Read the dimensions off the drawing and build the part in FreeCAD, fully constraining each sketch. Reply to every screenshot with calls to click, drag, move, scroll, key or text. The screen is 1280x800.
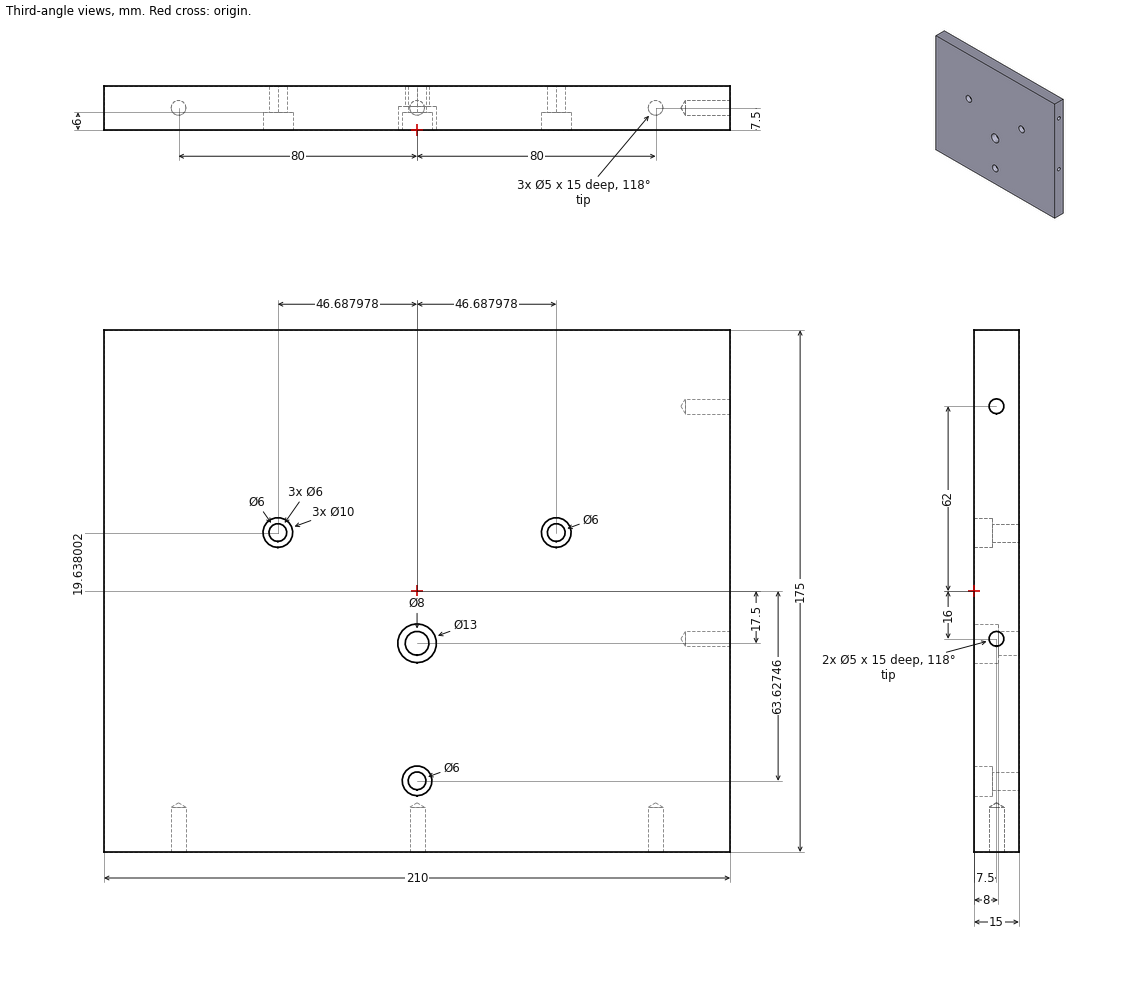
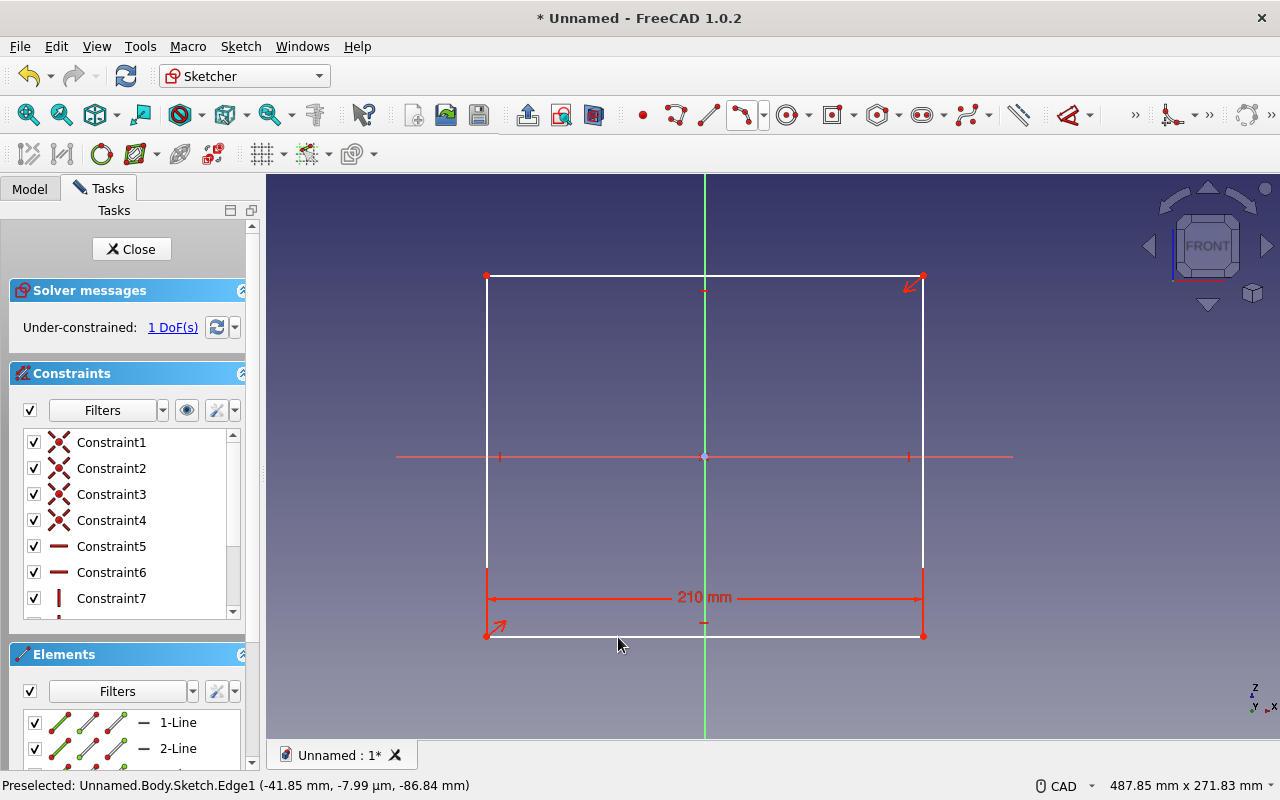
click(923, 529)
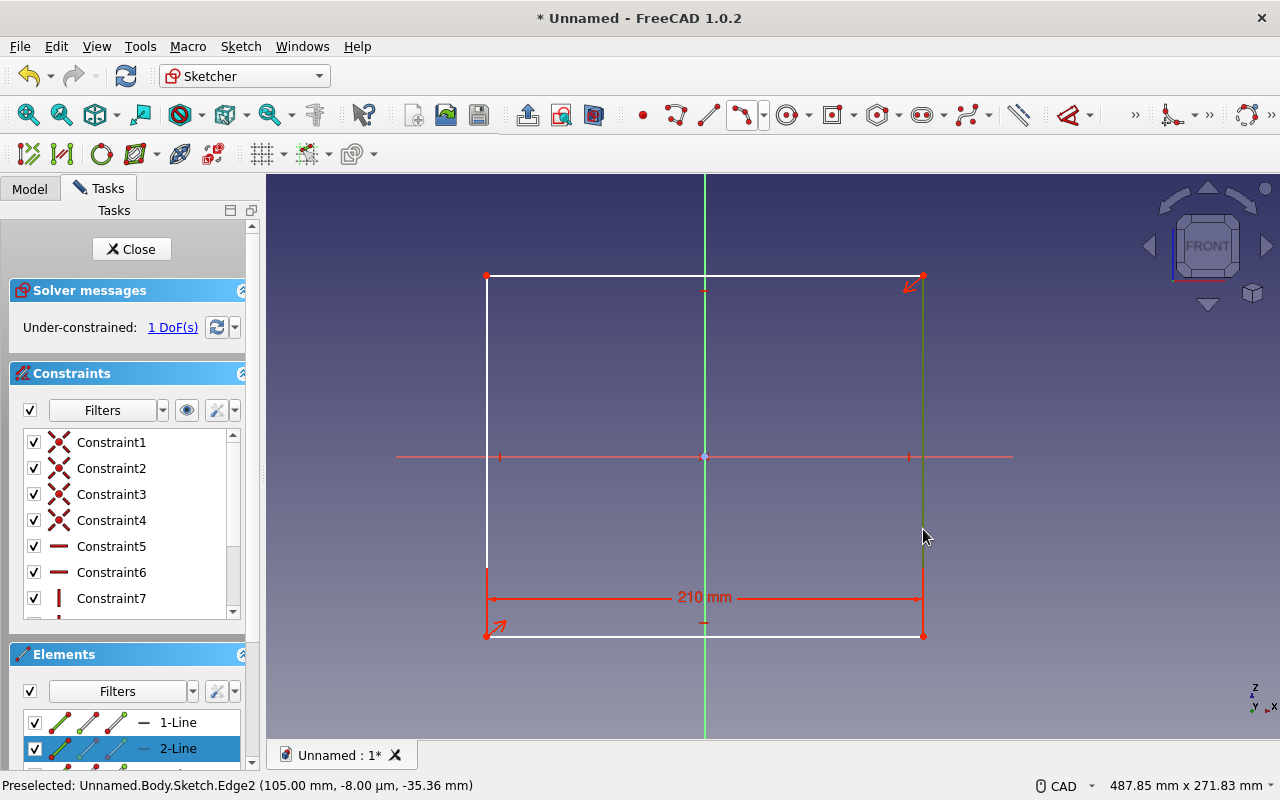
click(1090, 116)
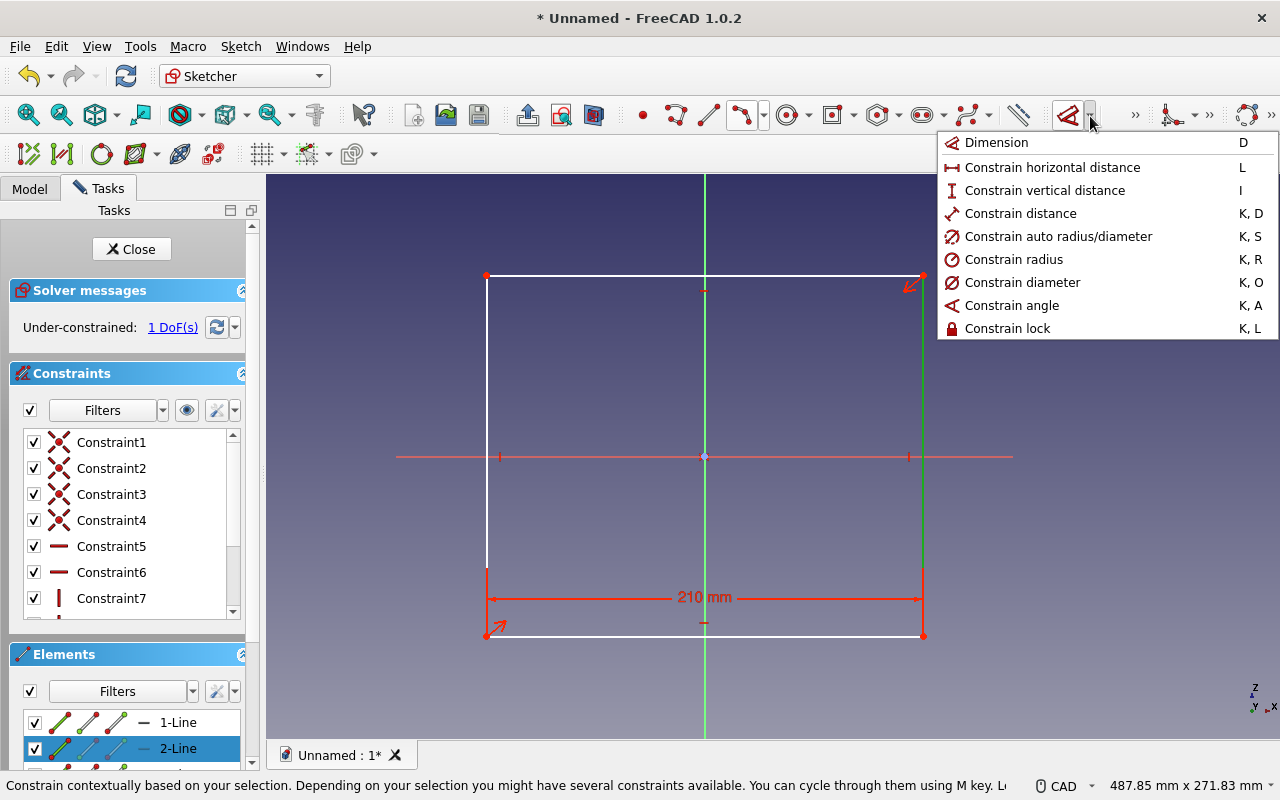
click(1108, 190)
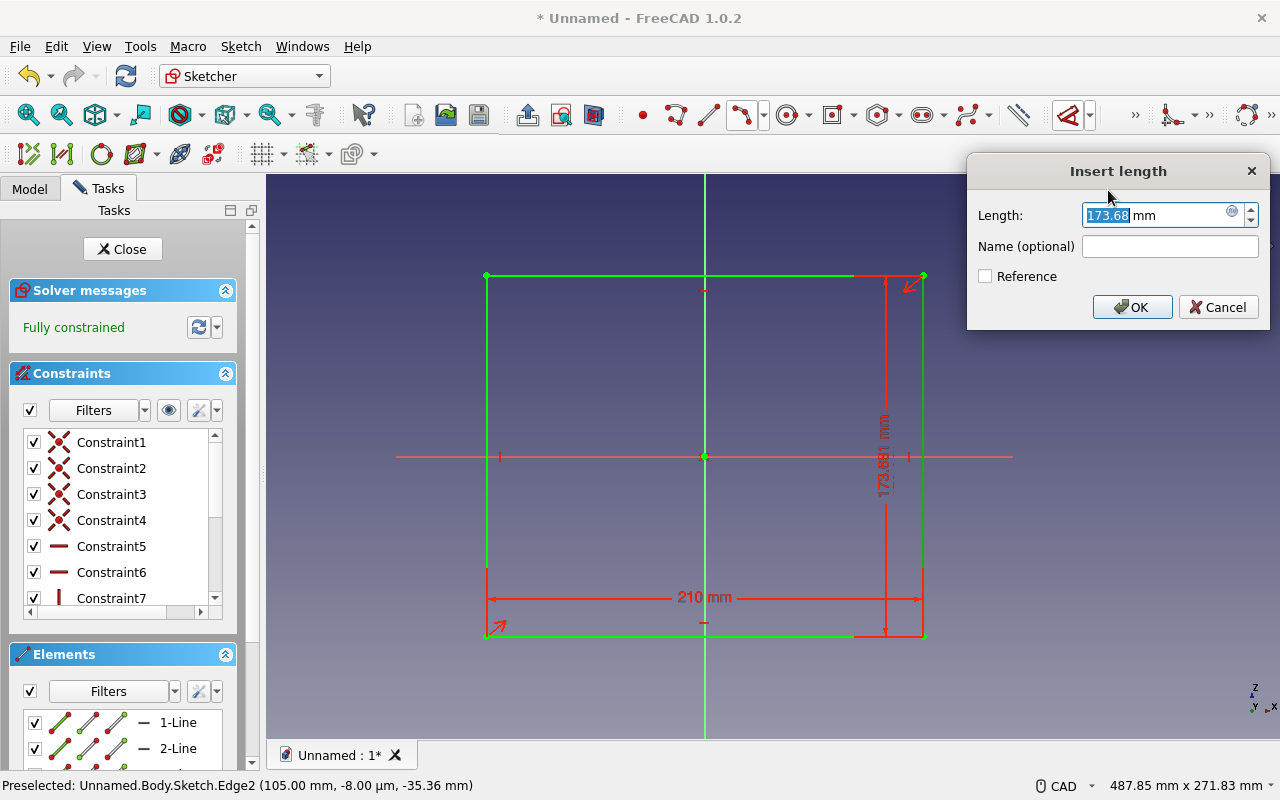
text(175)
key(Return)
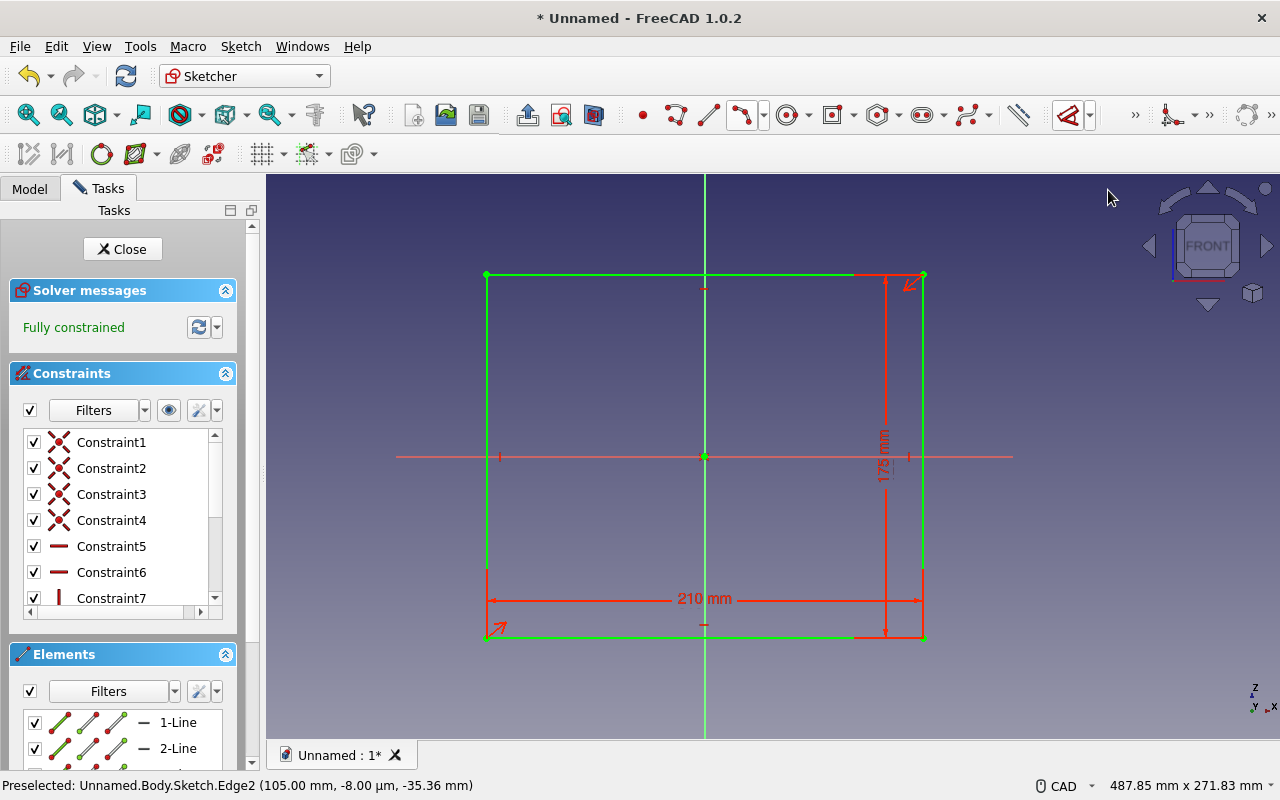
click(123, 249)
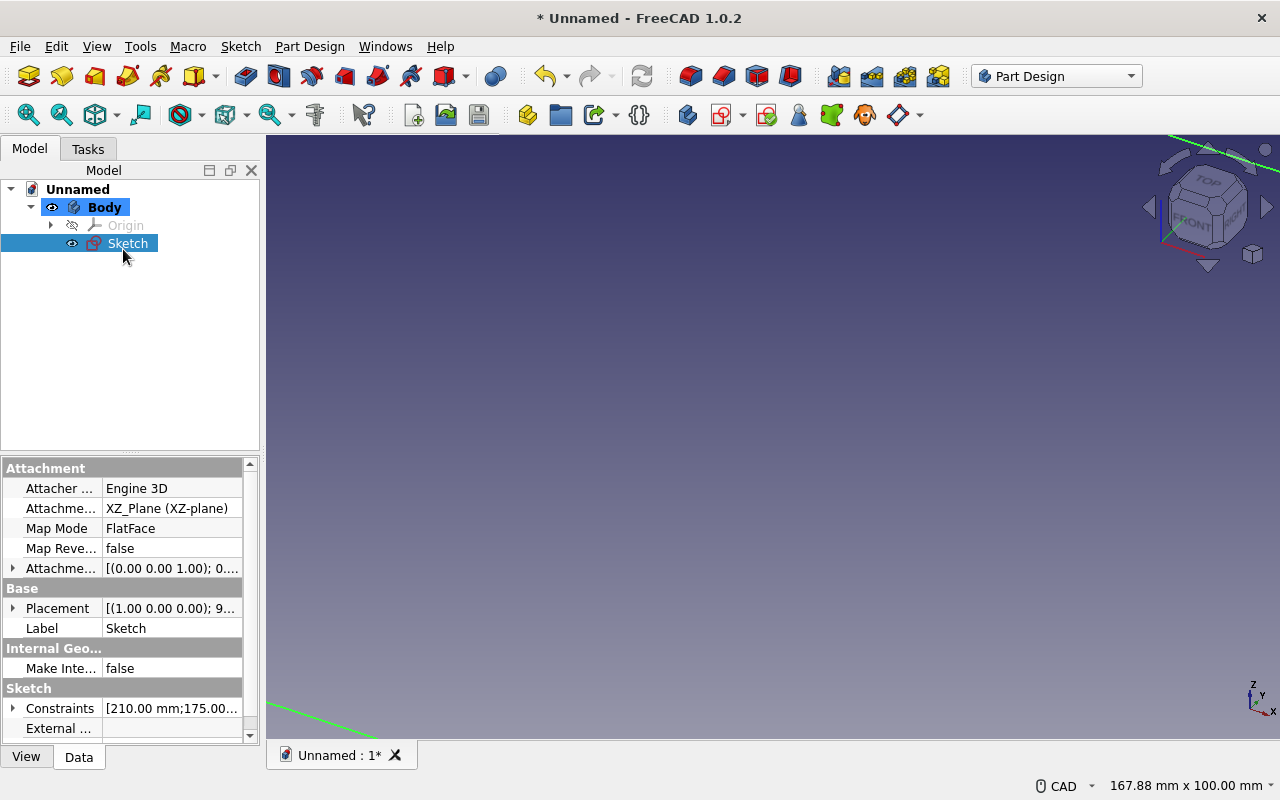
click(29, 76)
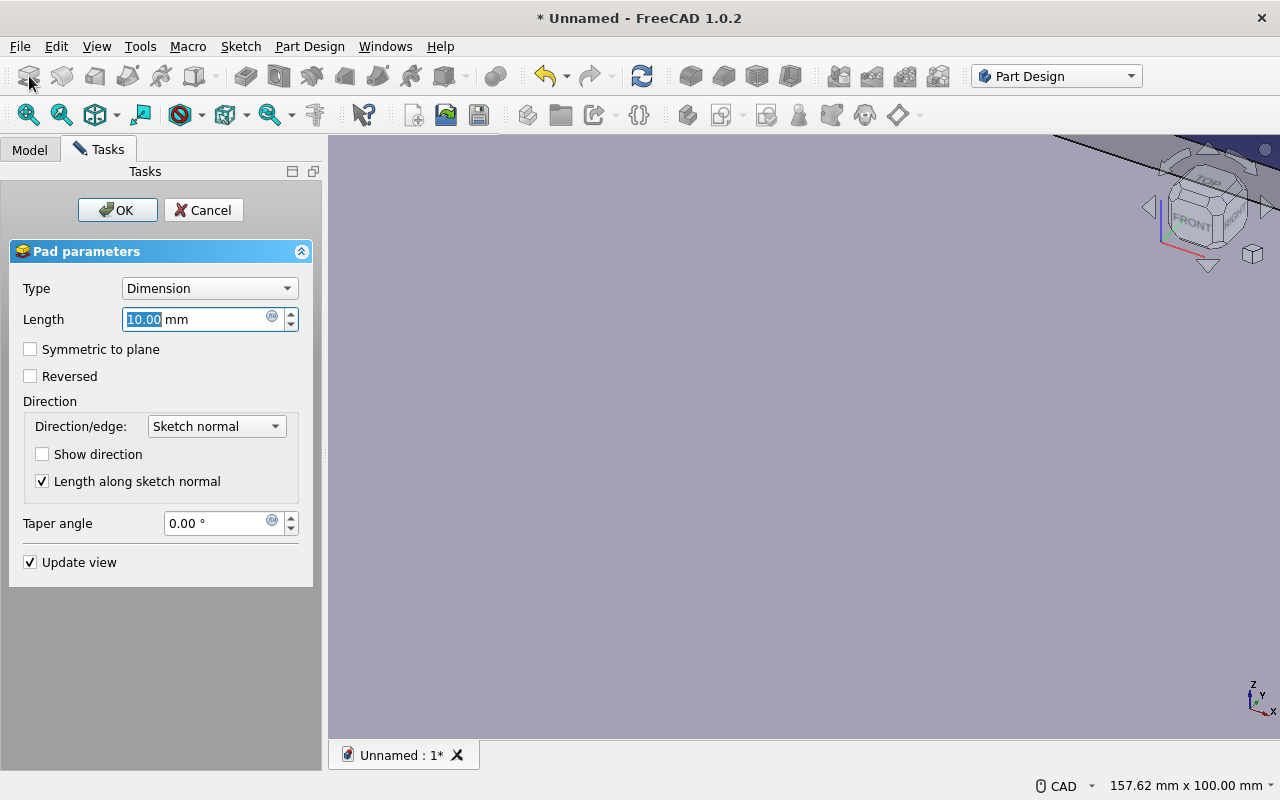
text(15)
key(Tab)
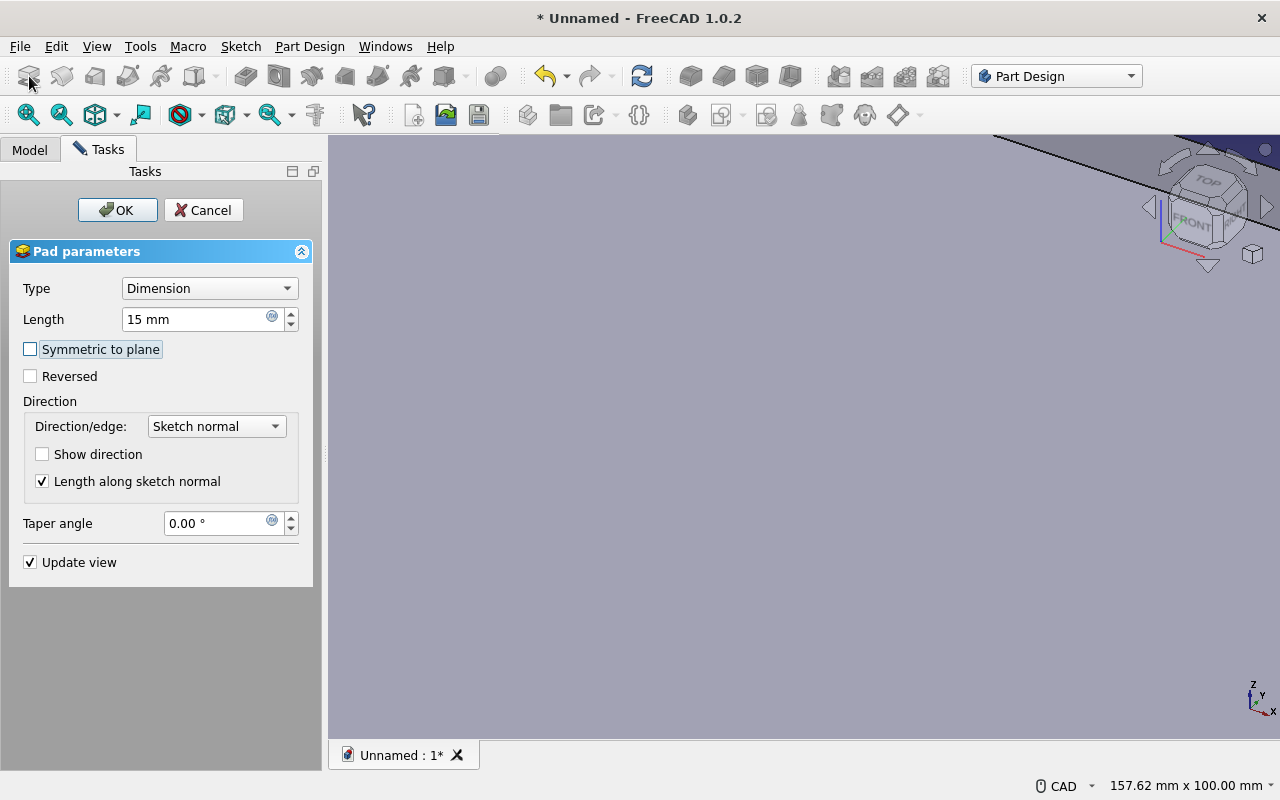
click(31, 376)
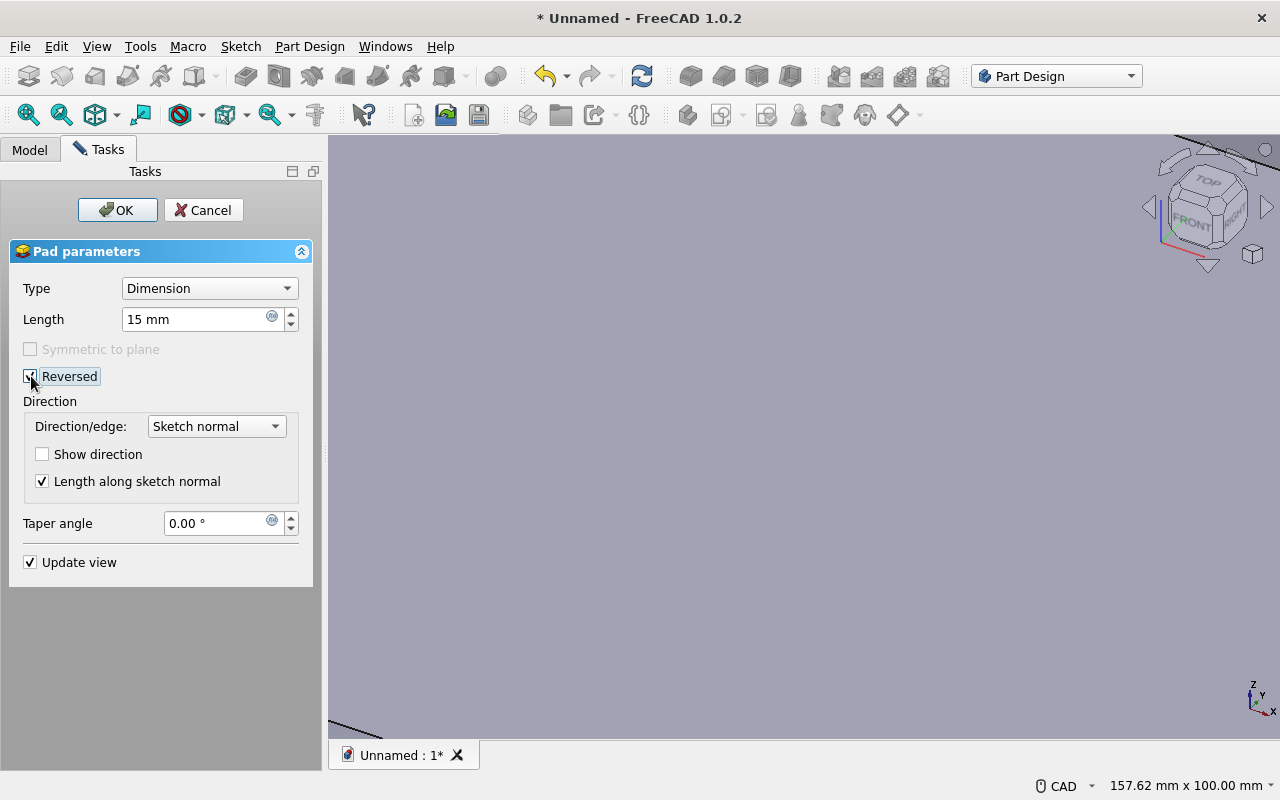
click(118, 210)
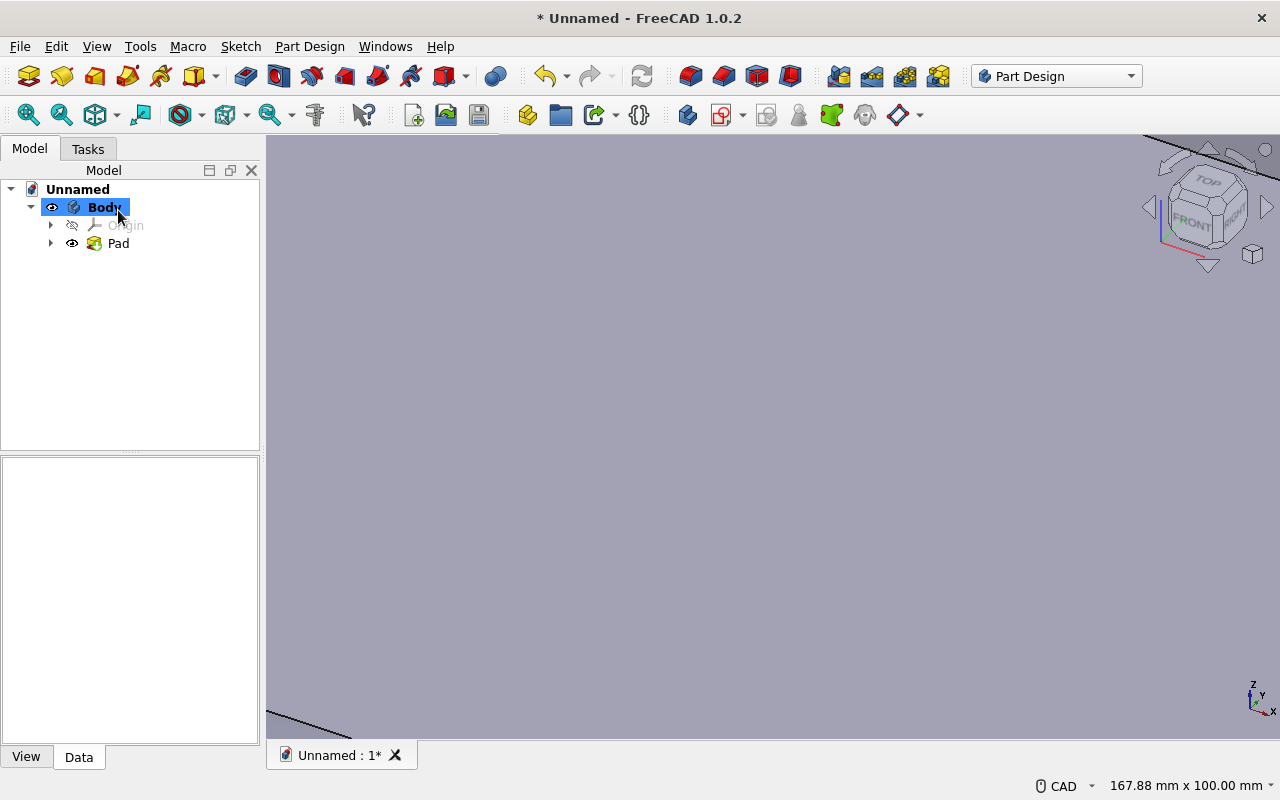
click(29, 116)